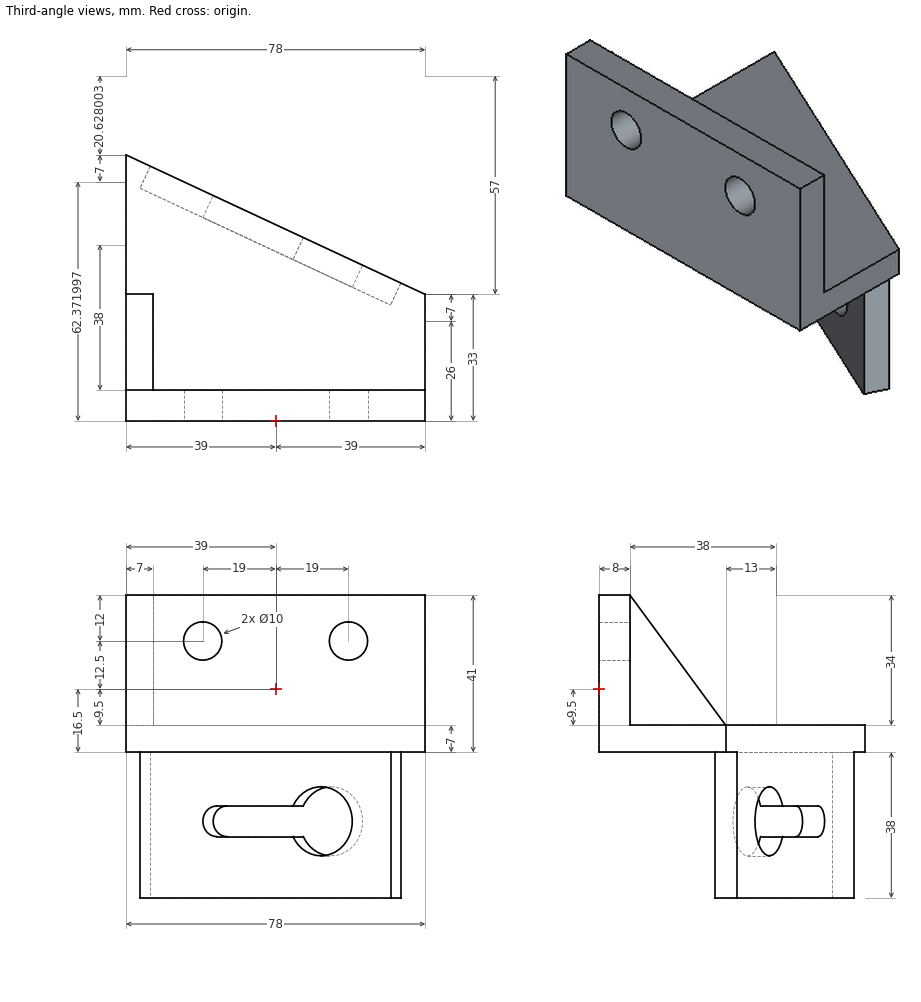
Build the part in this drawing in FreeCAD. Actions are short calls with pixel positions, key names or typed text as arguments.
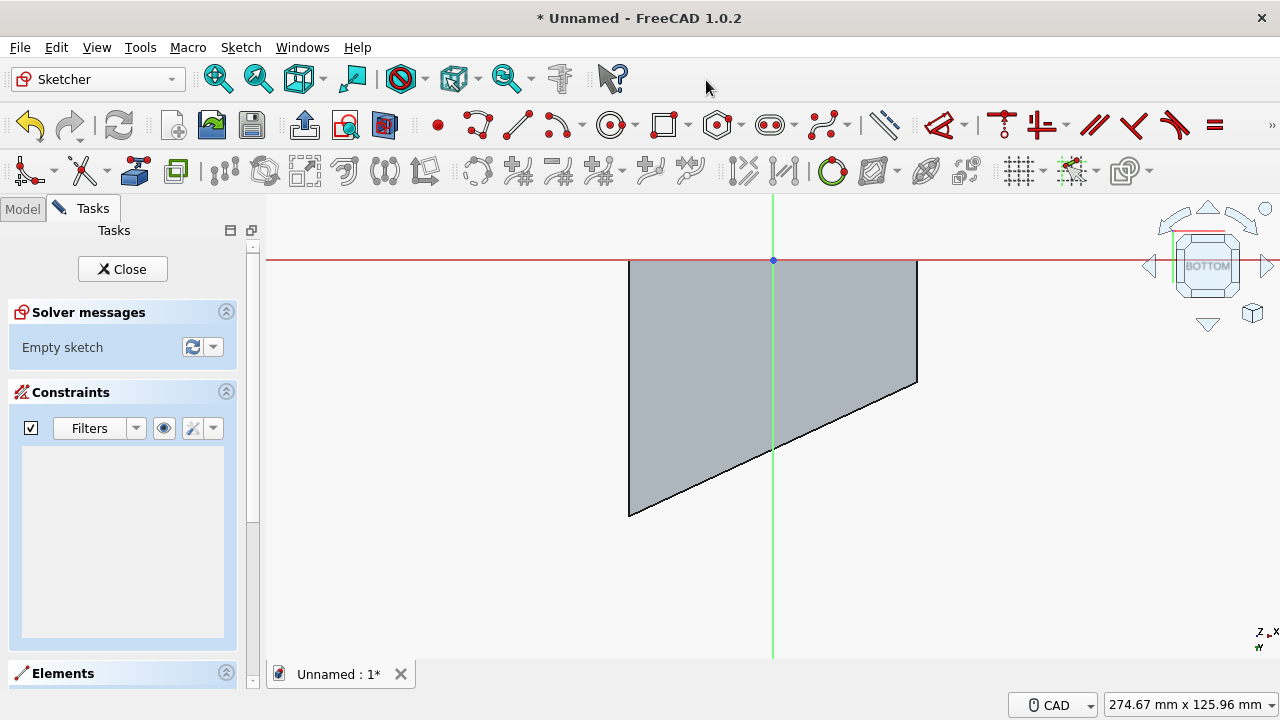
click(917, 356)
click(629, 491)
click(629, 516)
click(917, 382)
click(917, 357)
key(Escape)
key(Escape)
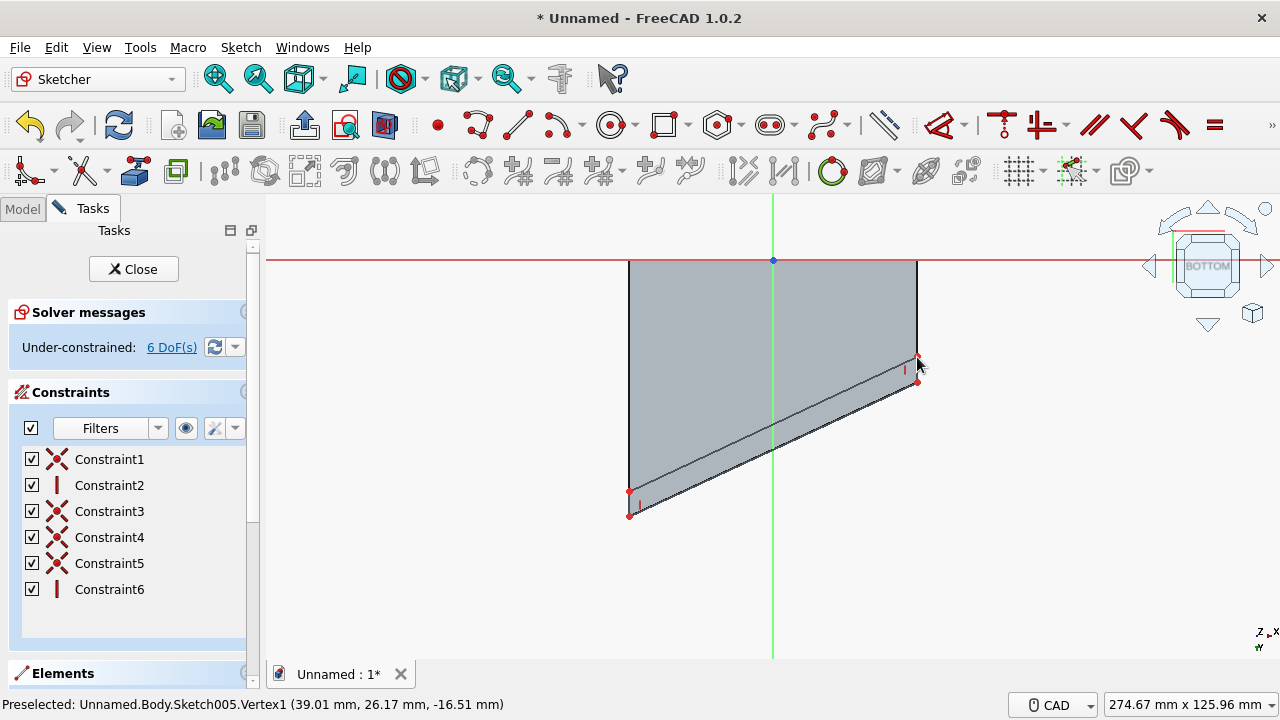
click(940, 126)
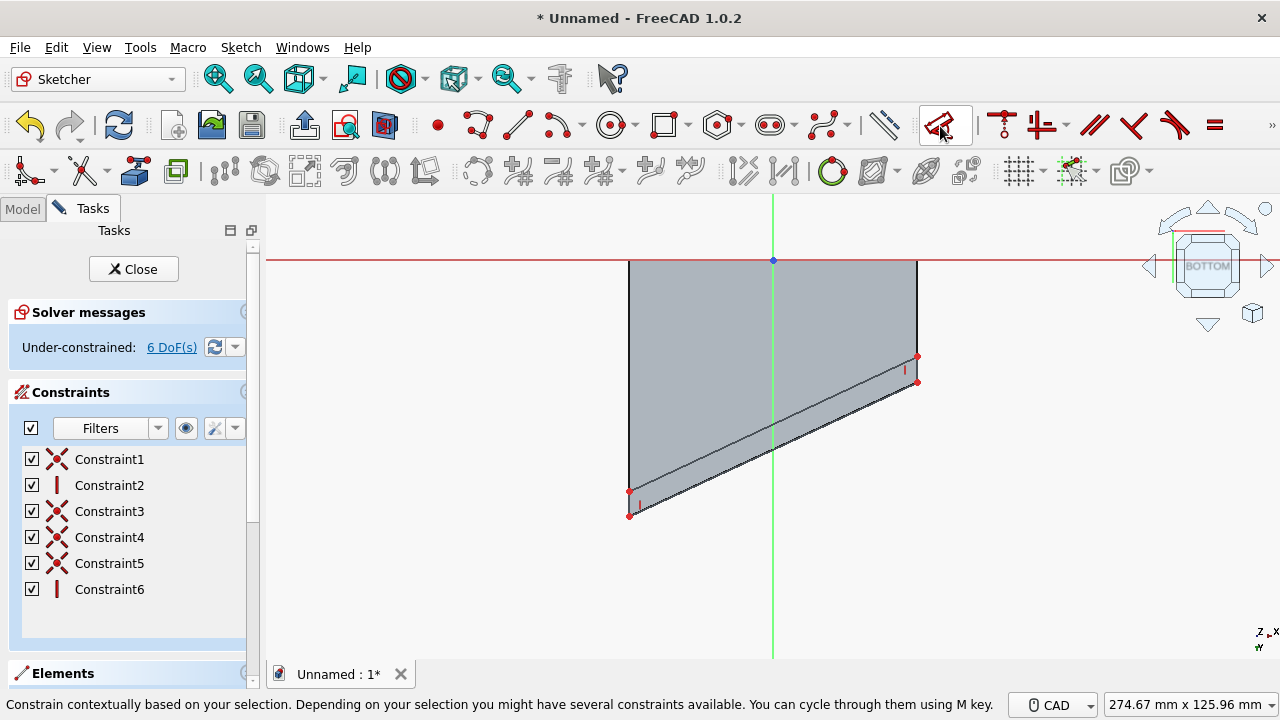
scroll(629, 502, up, 3)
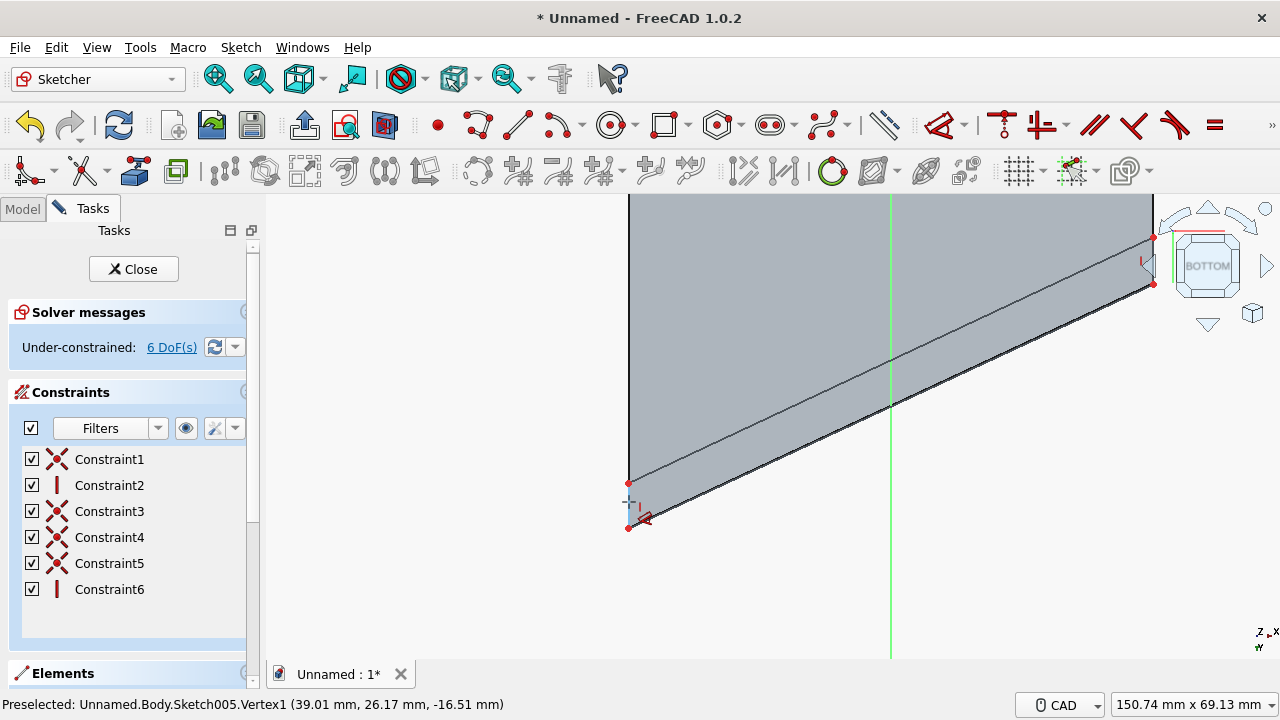
click(629, 501)
click(595, 506)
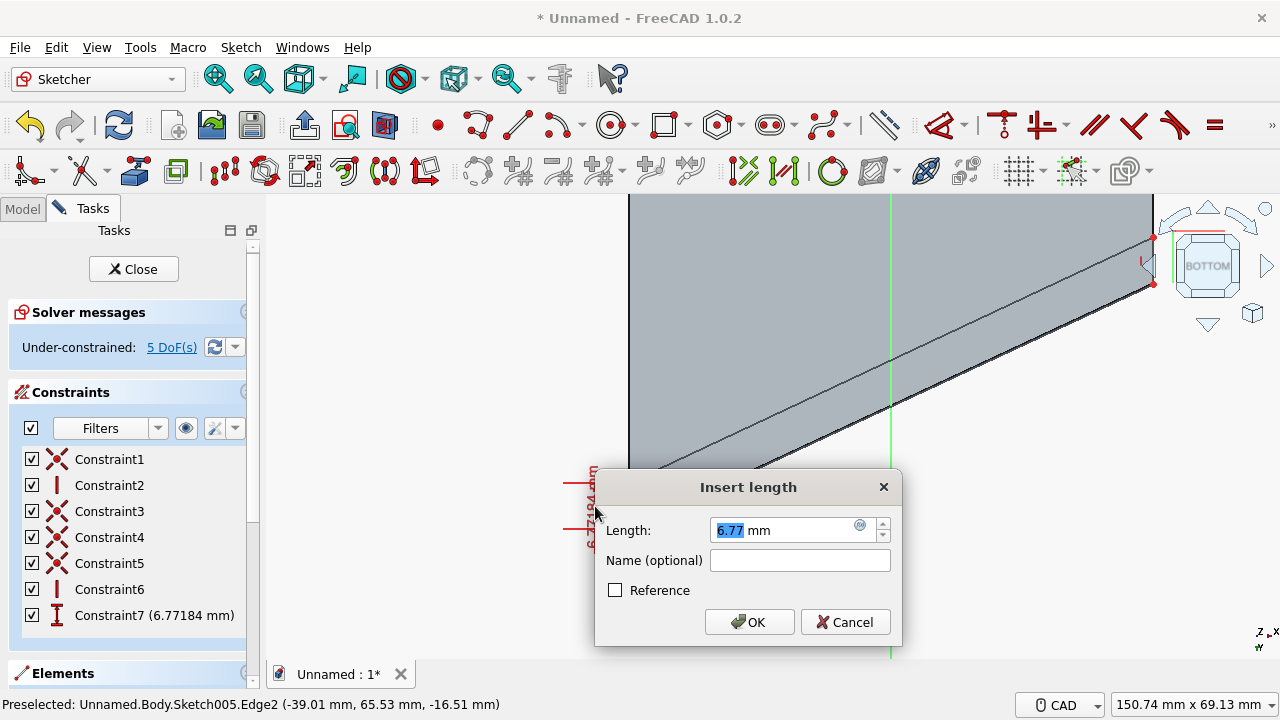
text(7)
key(Return)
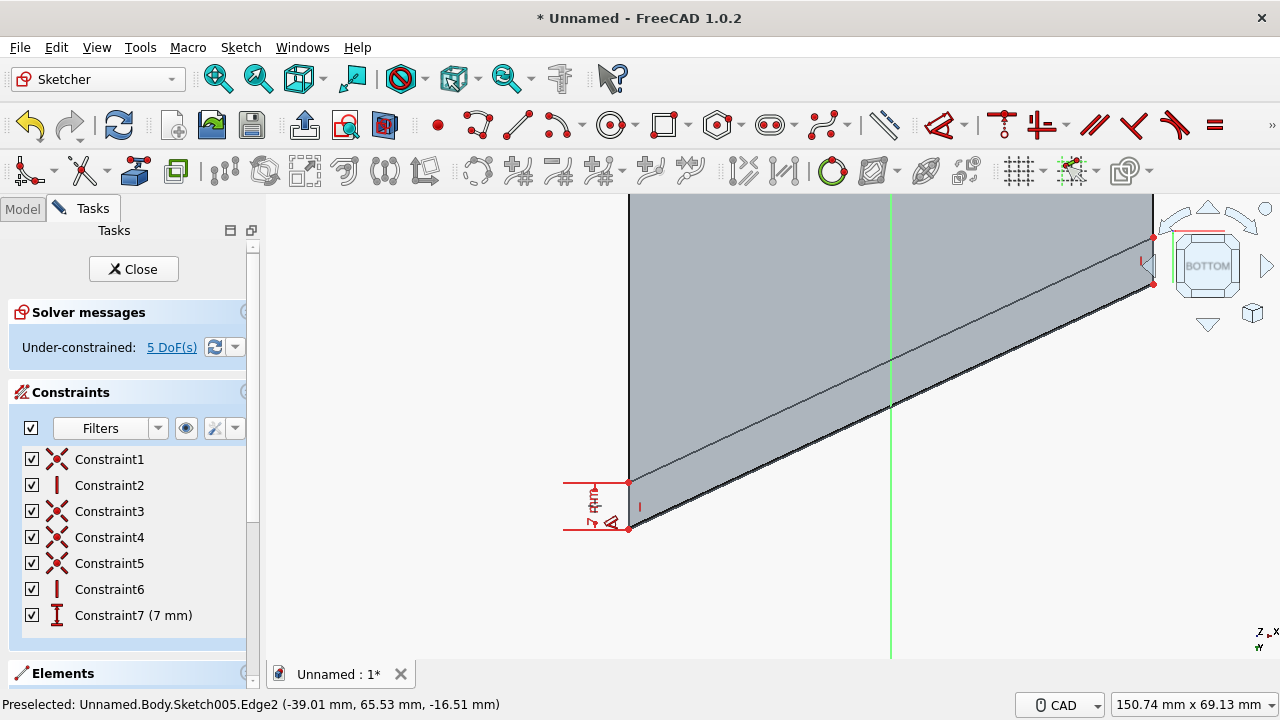
scroll(325, 631, down, 2)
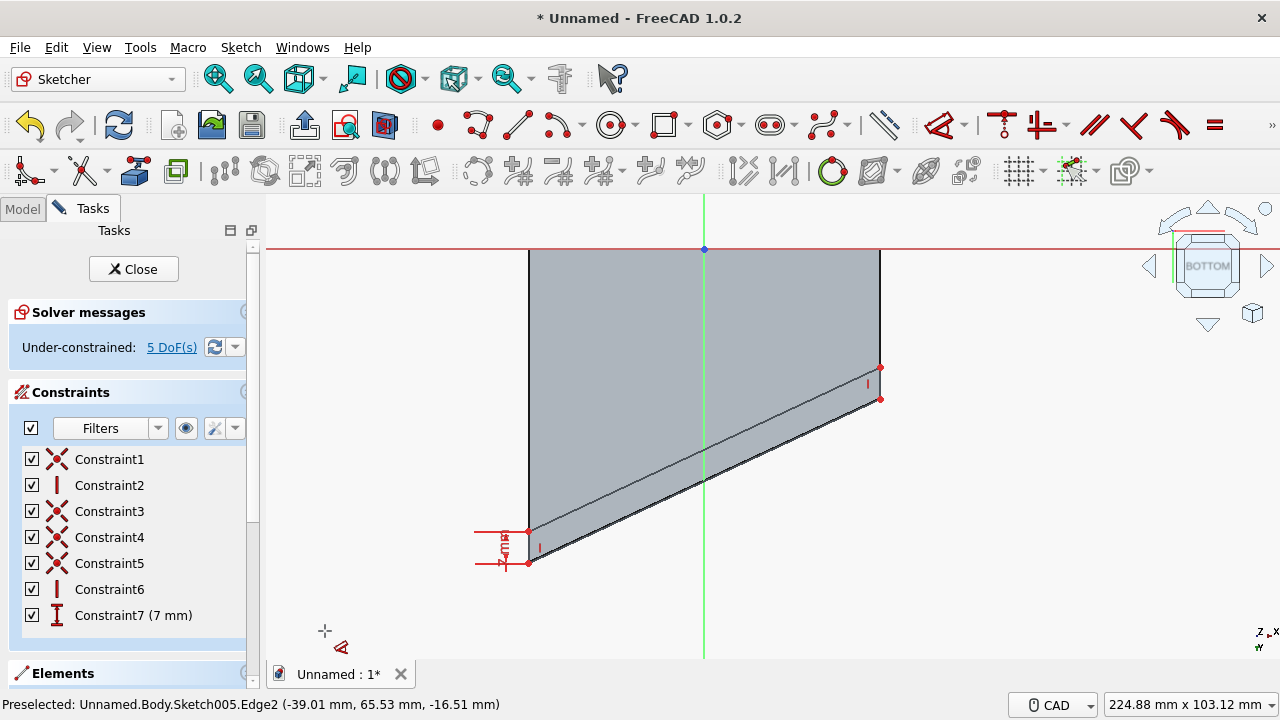
scroll(880, 390, up, 2)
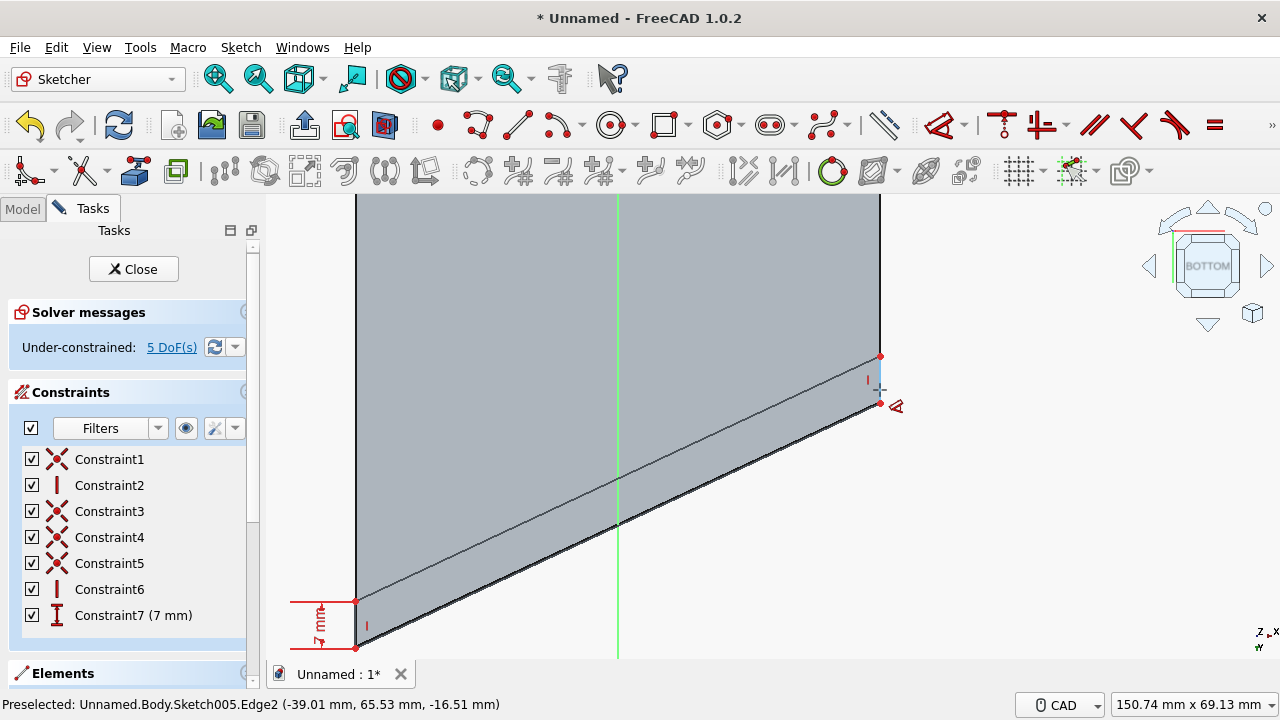
click(880, 389)
click(914, 380)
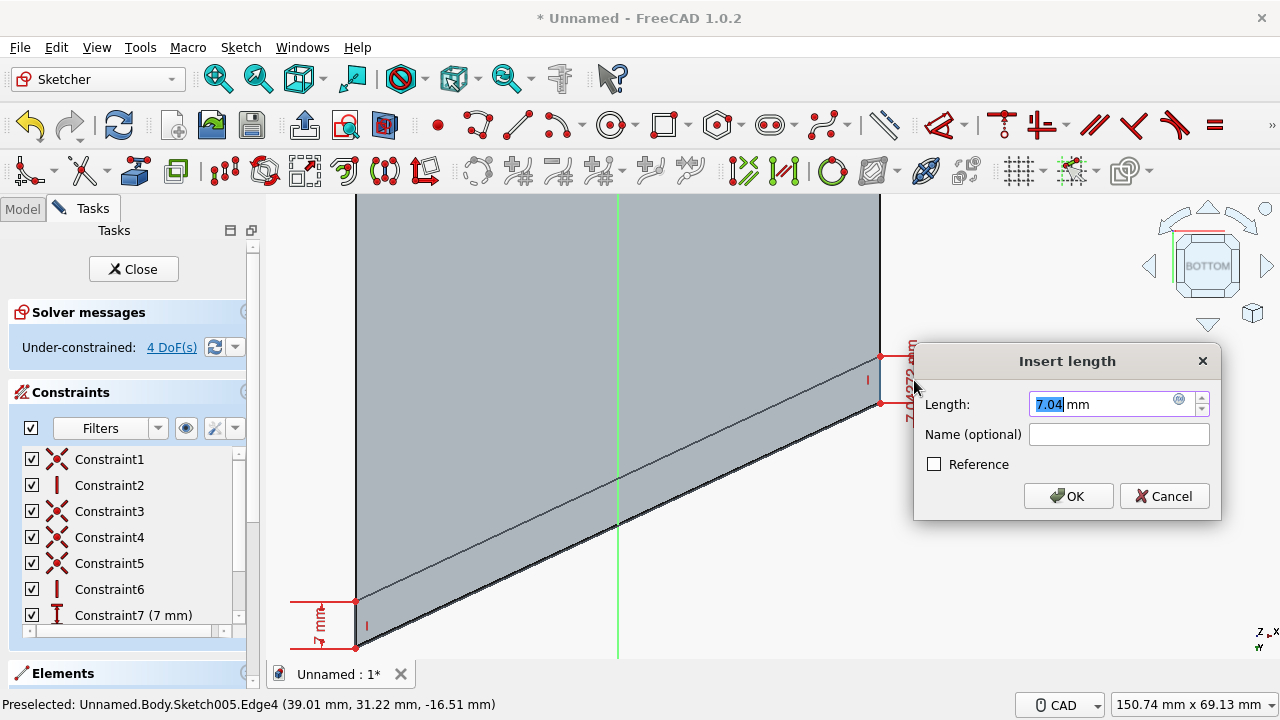
text(7)
key(Return)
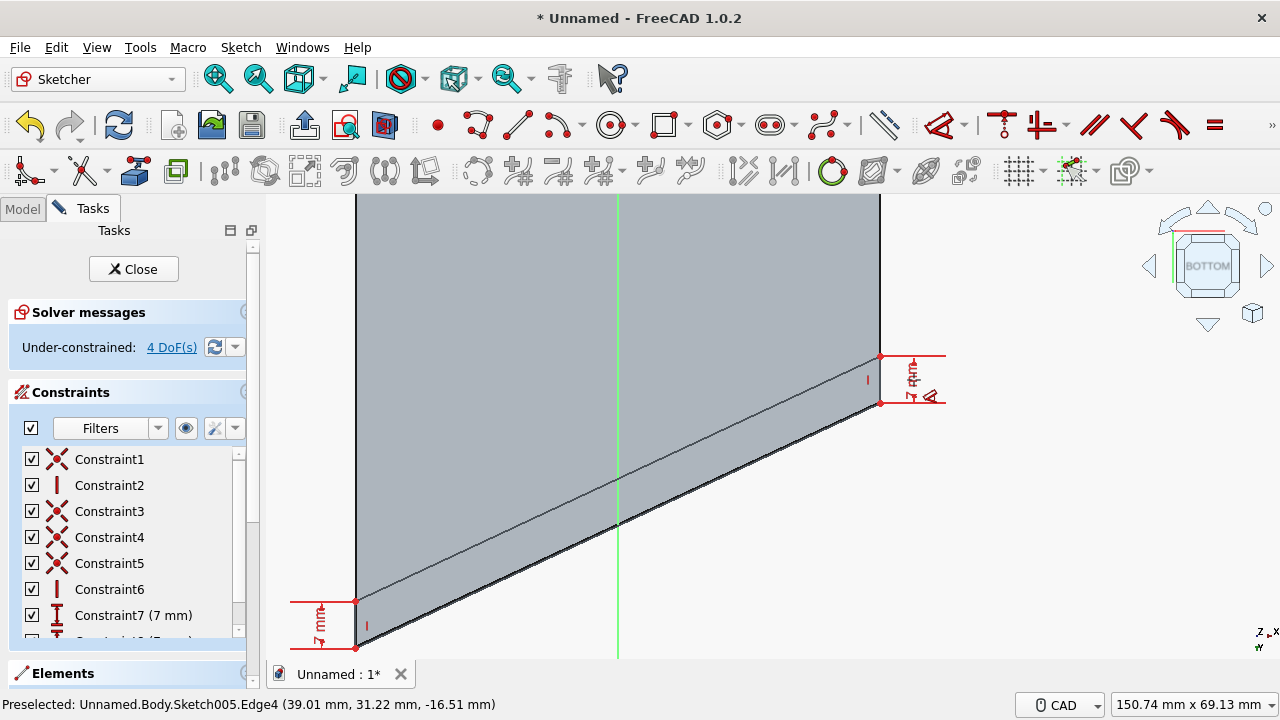
click(880, 356)
click(749, 390)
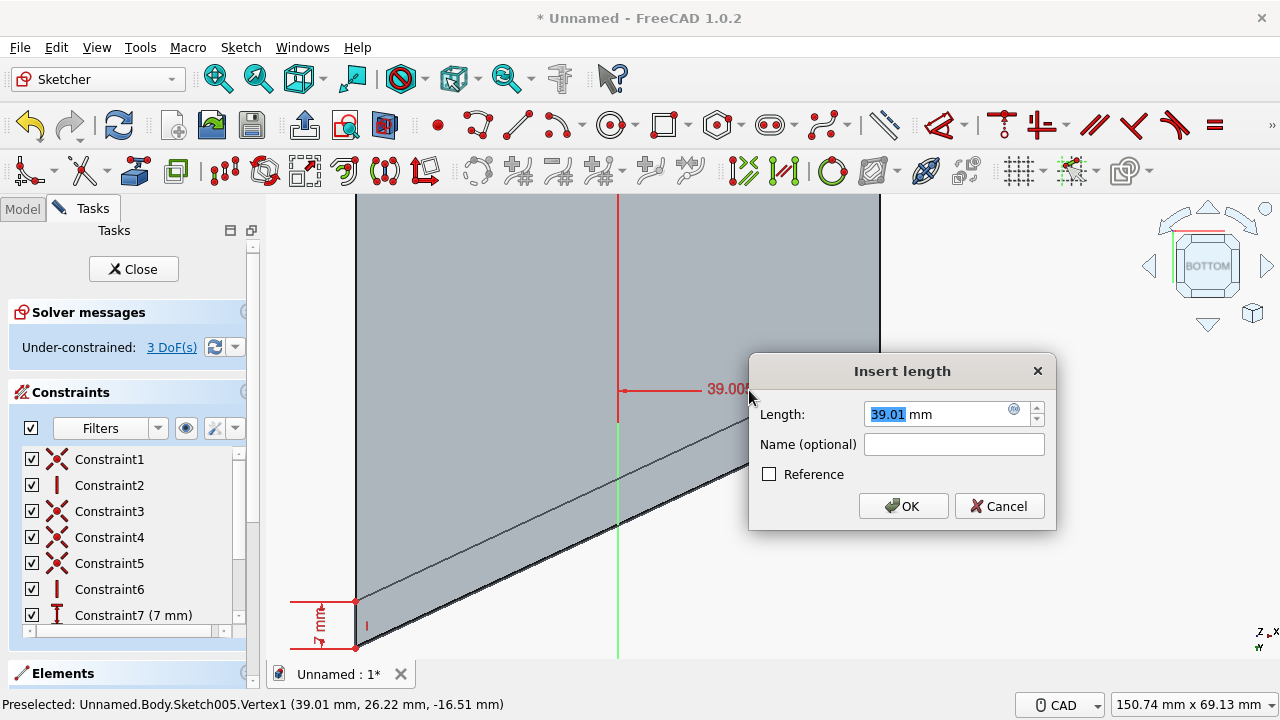
text(39)
key(Return)